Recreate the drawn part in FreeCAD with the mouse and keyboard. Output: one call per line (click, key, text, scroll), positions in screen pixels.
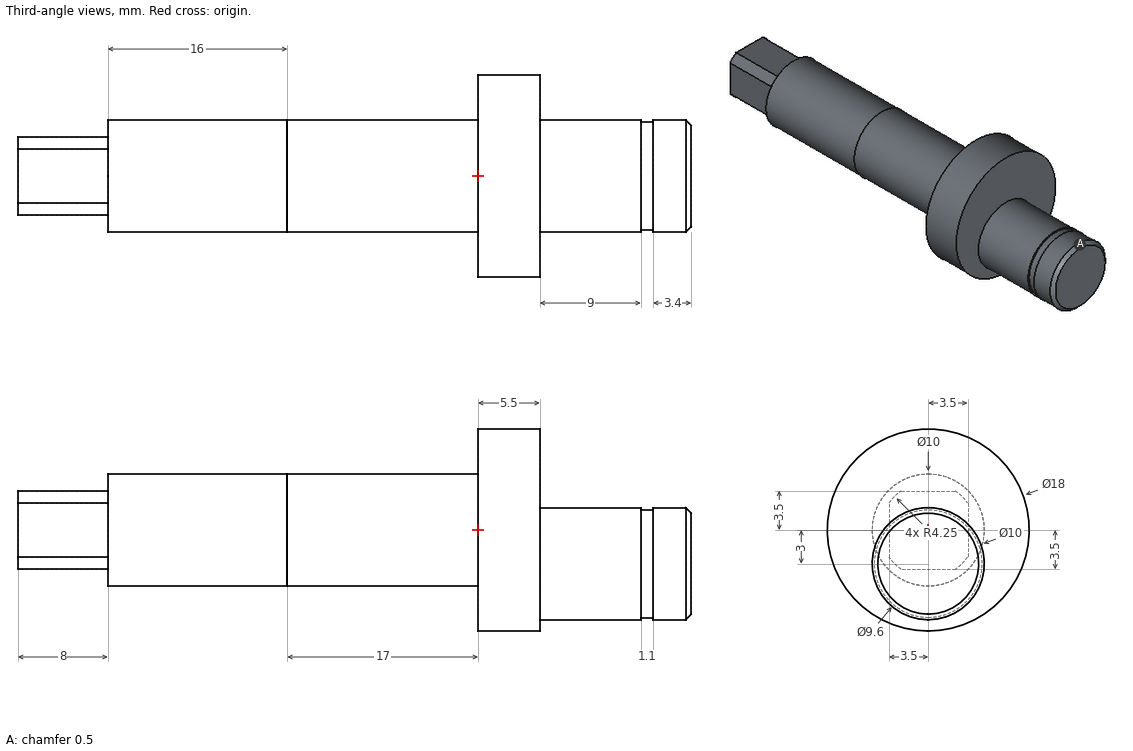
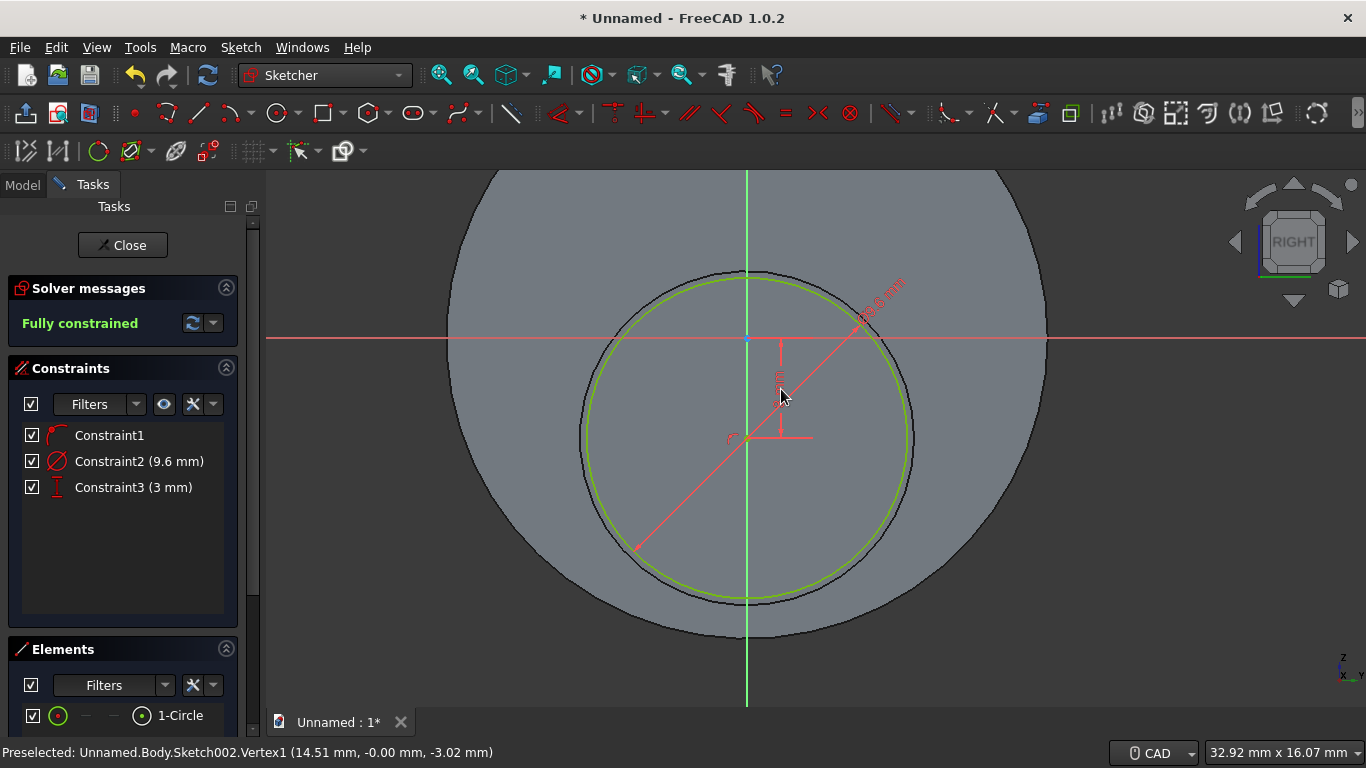
click(123, 245)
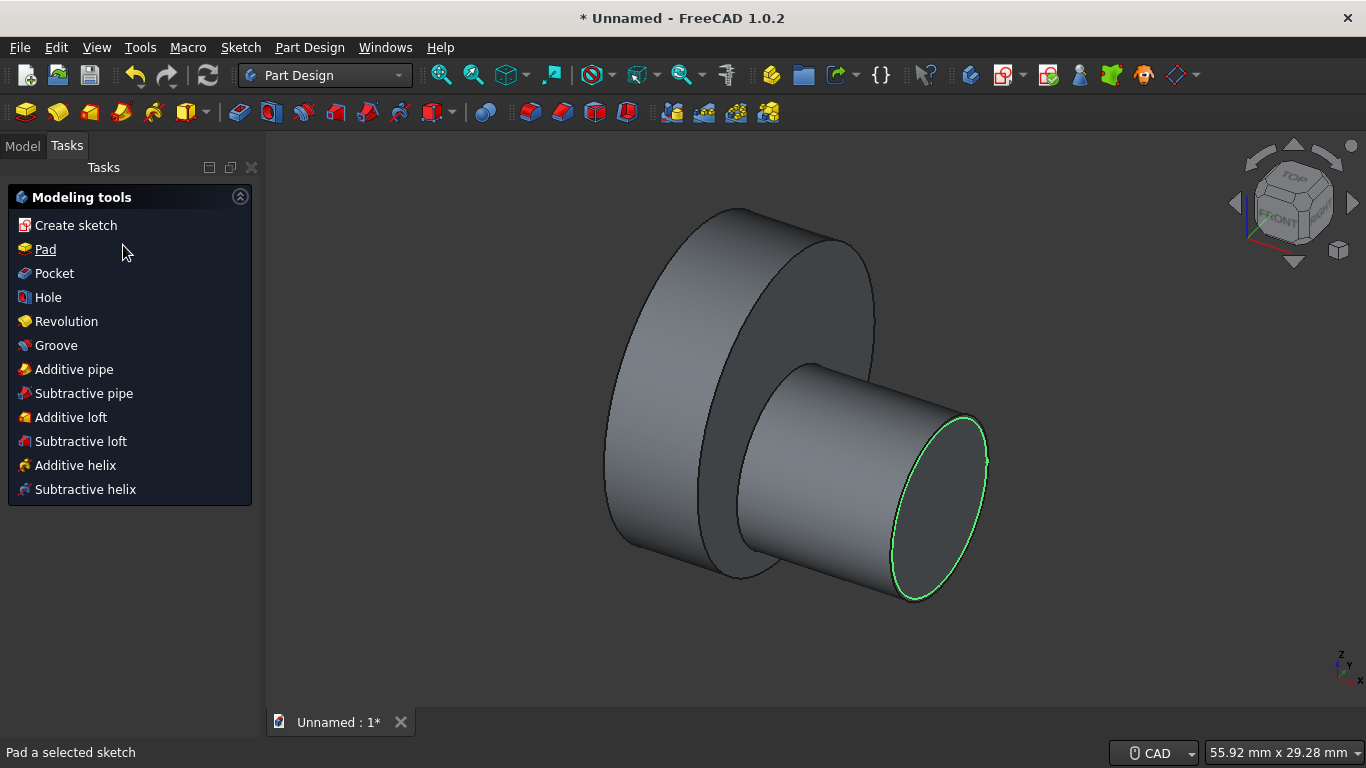
click(26, 112)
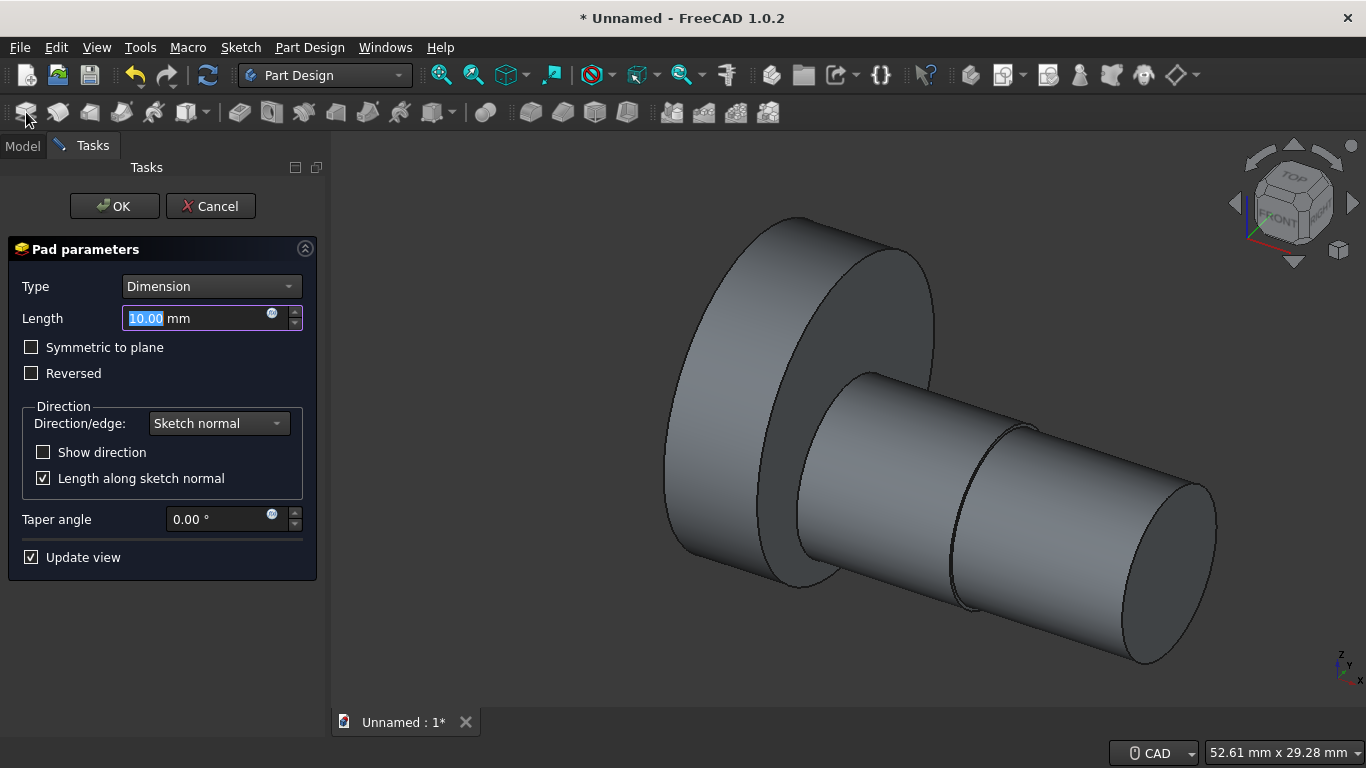
text(1.1)
key(Tab)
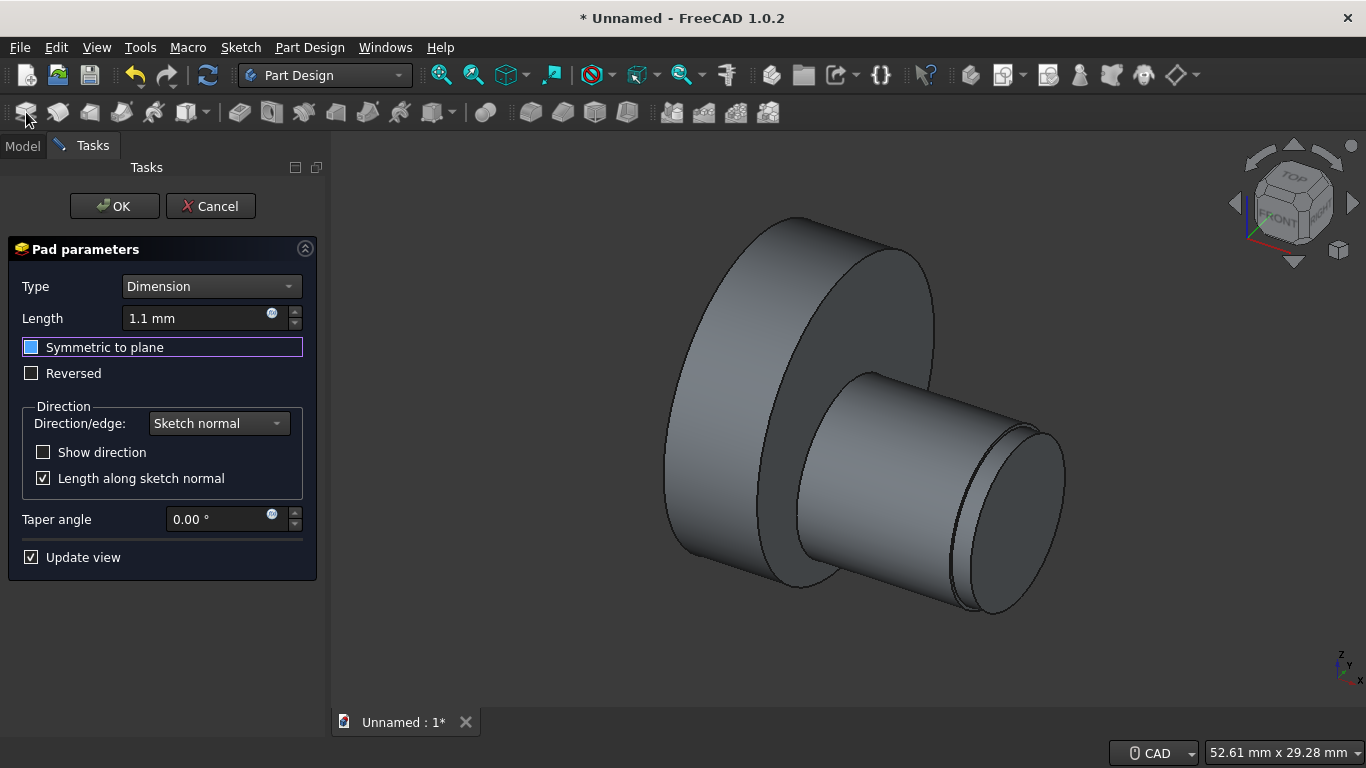
click(115, 206)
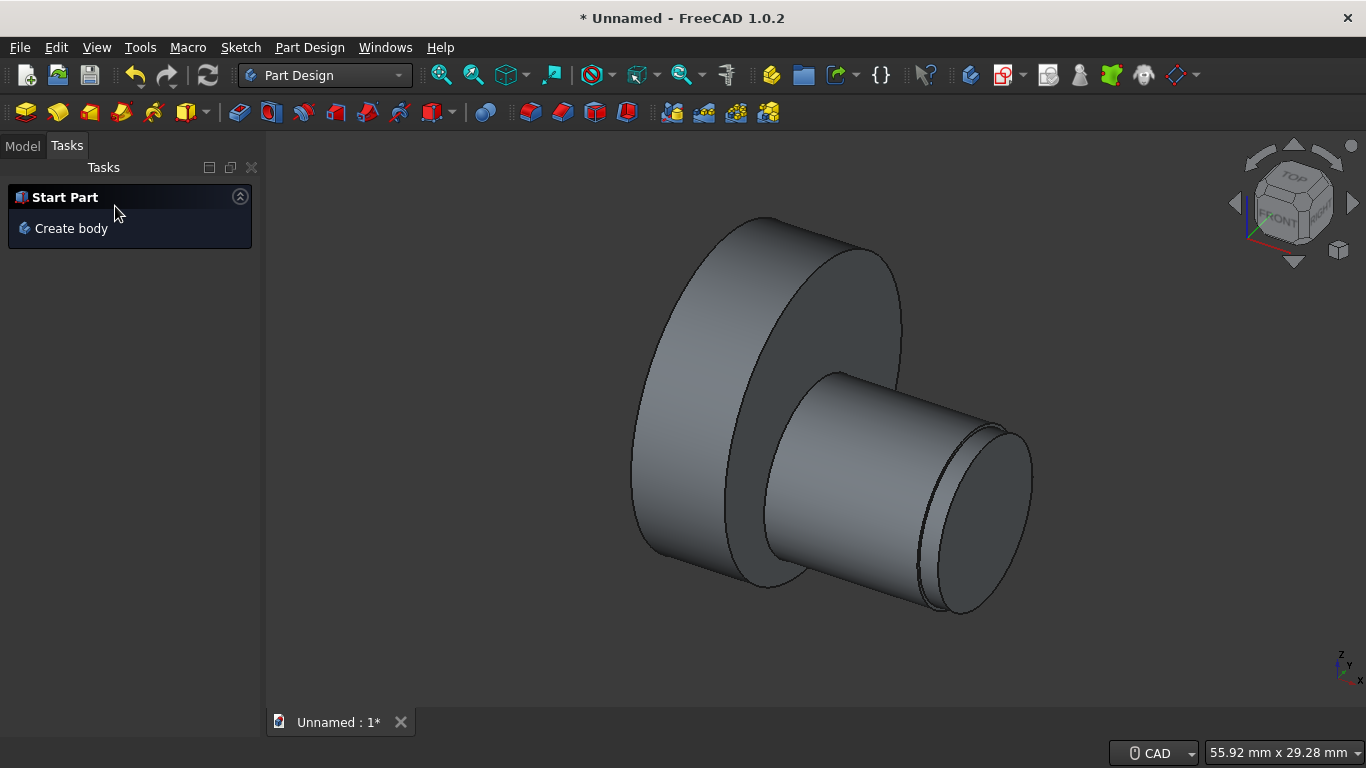
click(985, 523)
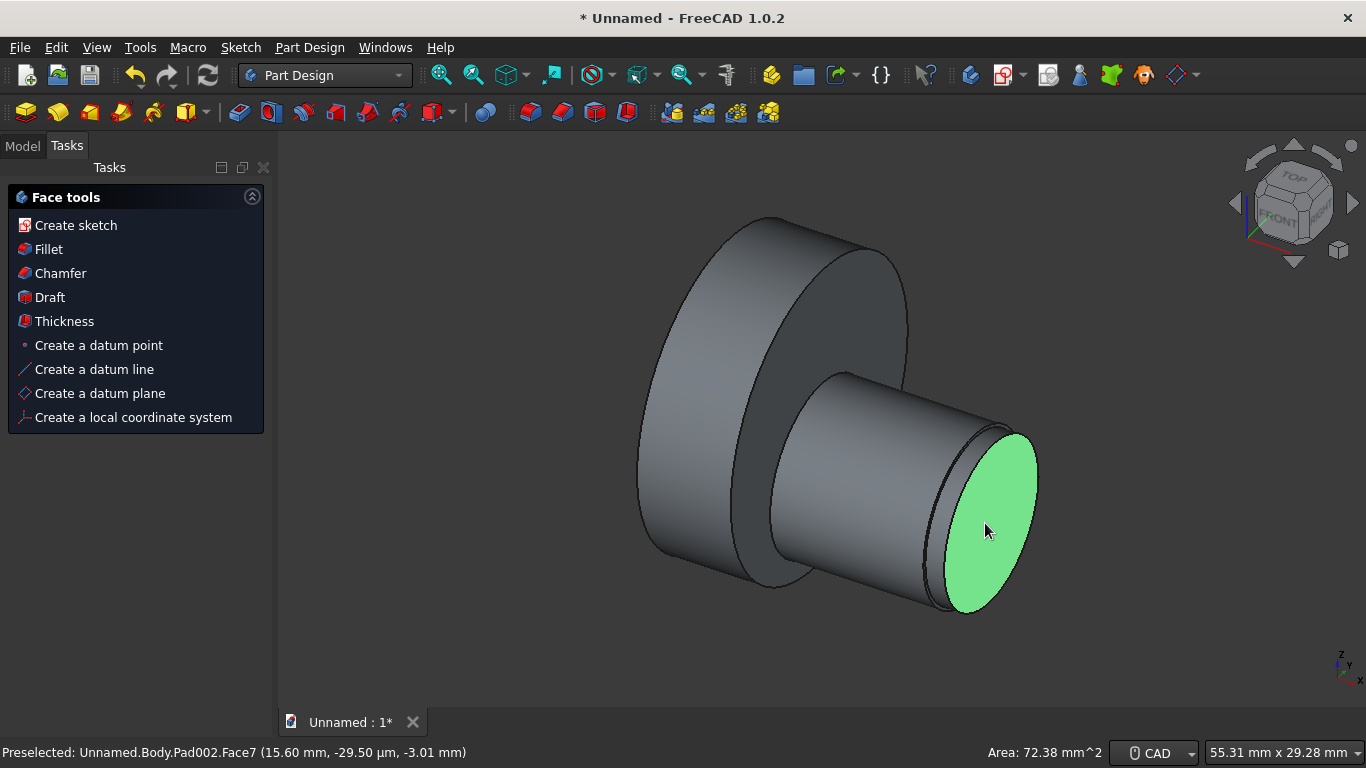
click(1004, 76)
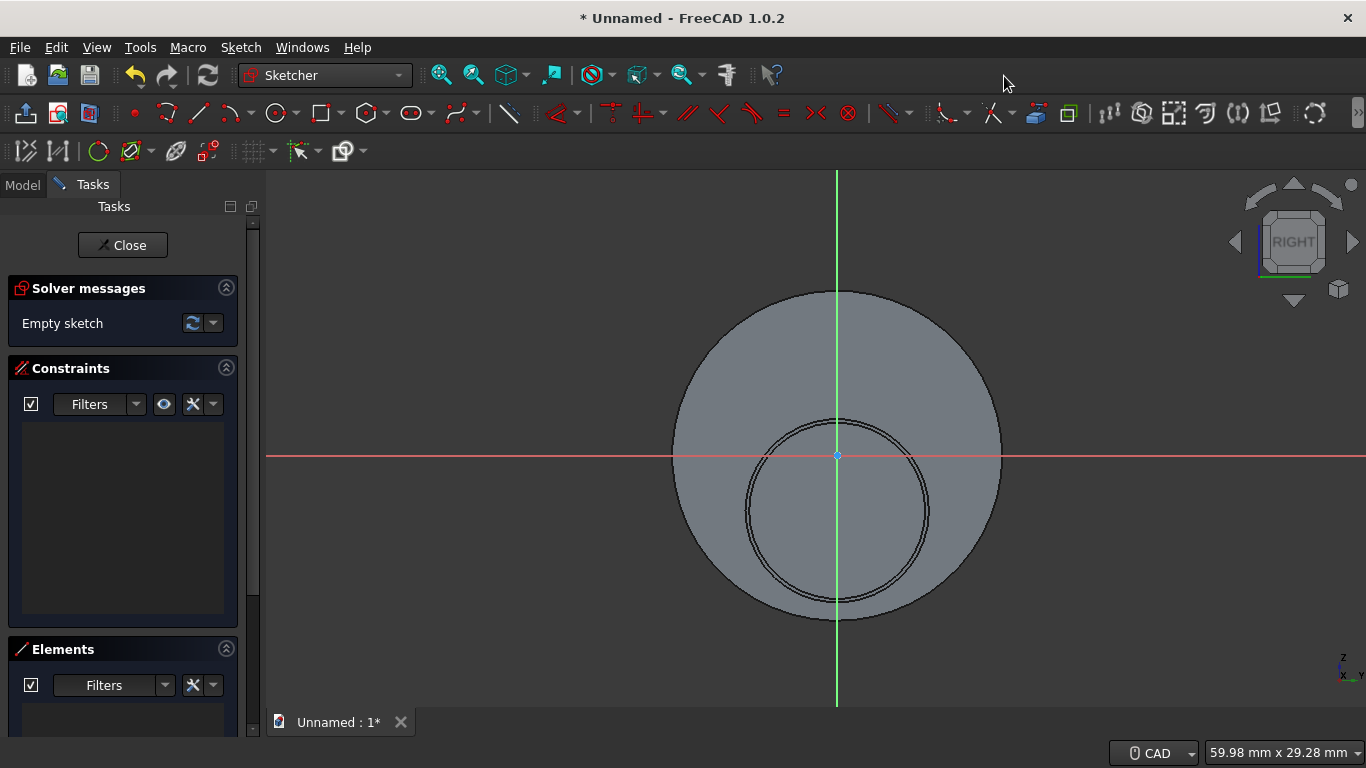
scroll(946, 599, up, 3)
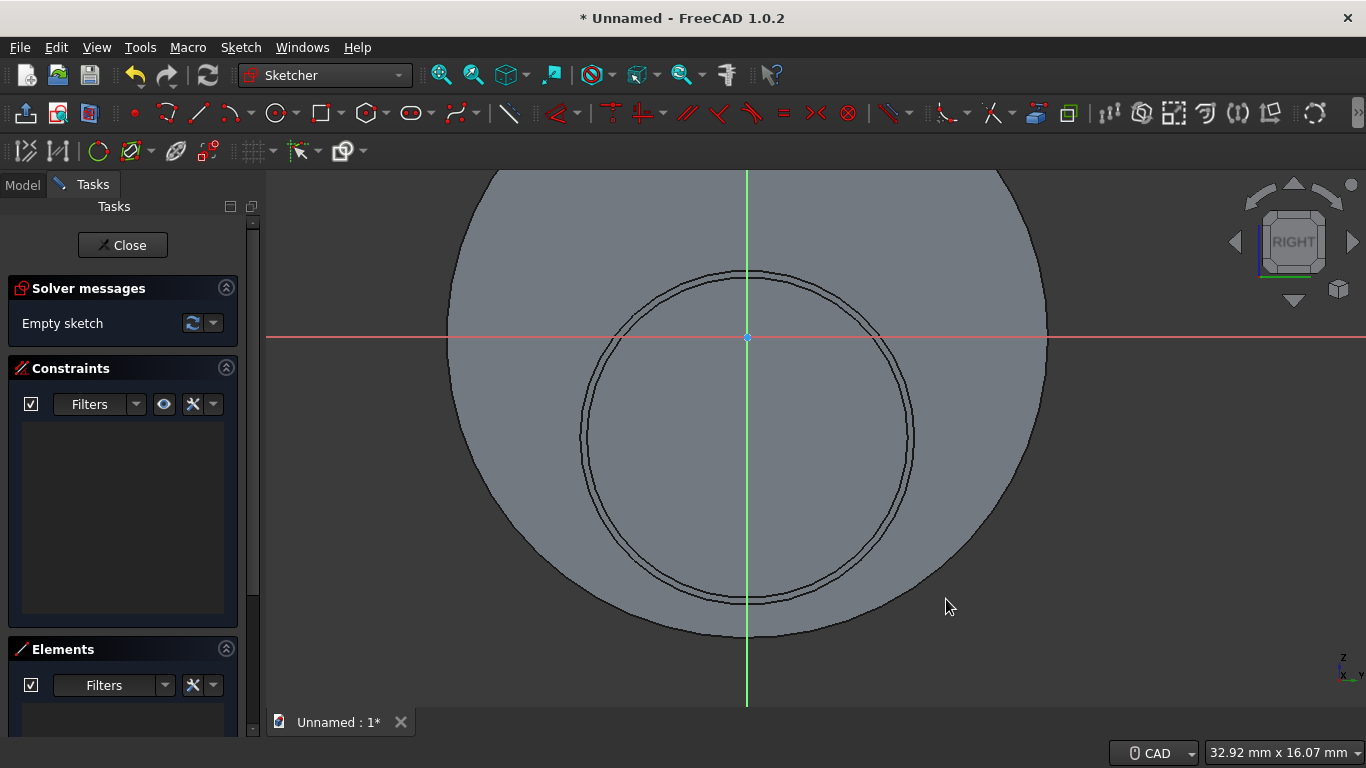
key(g)
key(c)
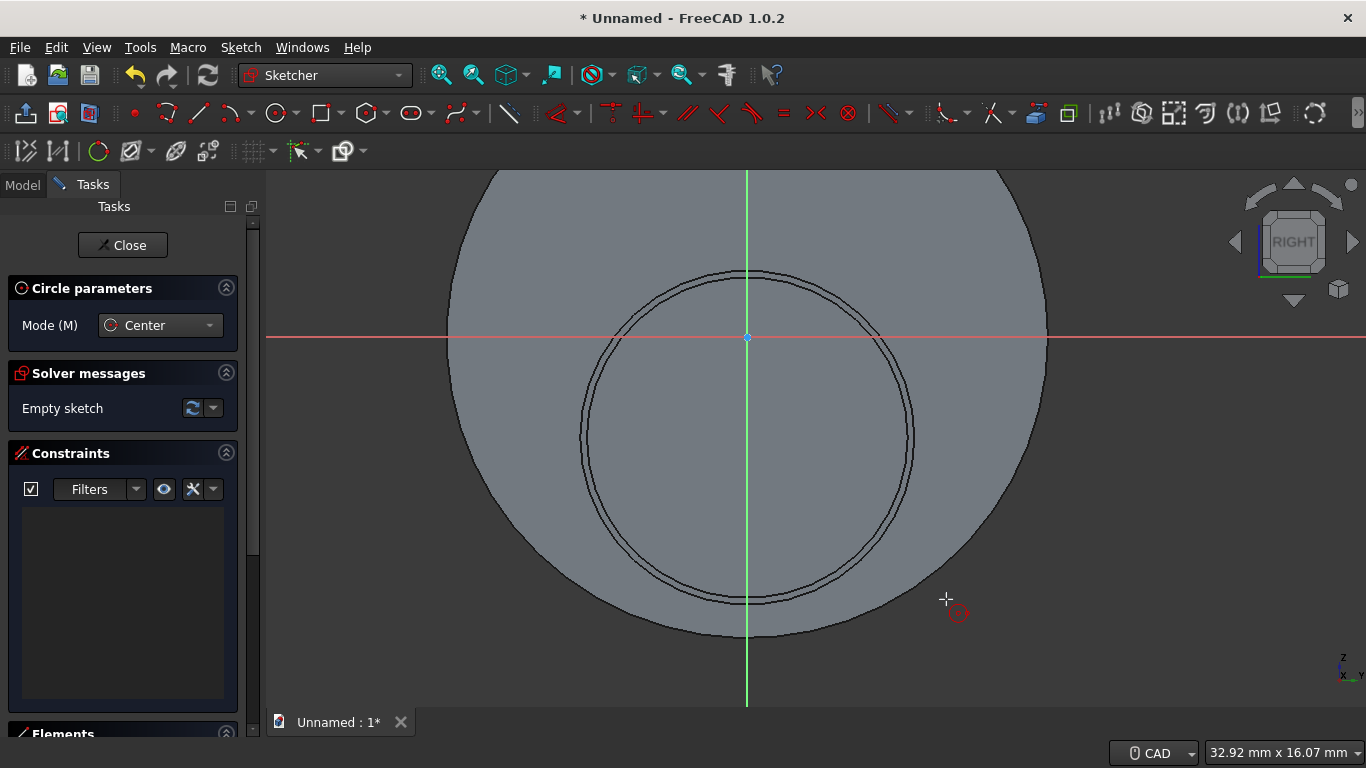
click(747, 438)
click(865, 319)
key(Escape)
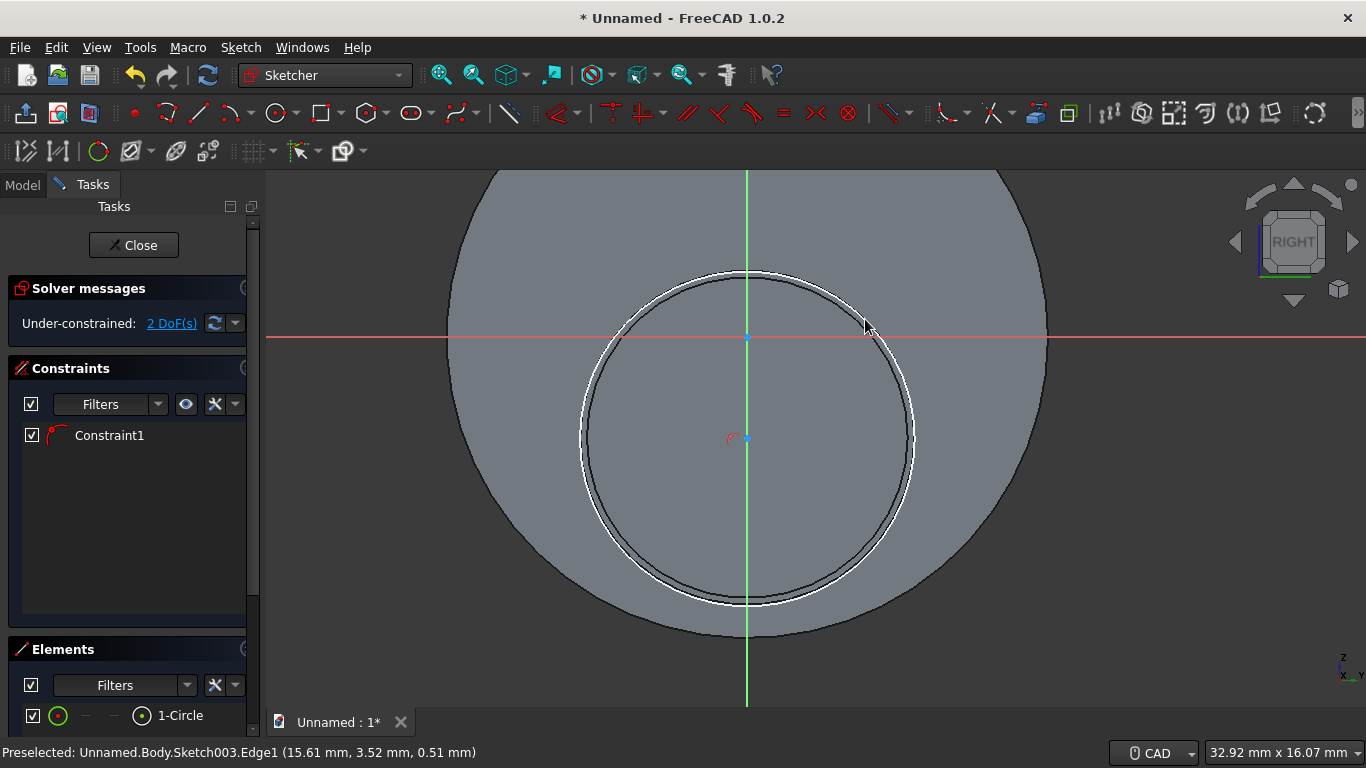
key(d)